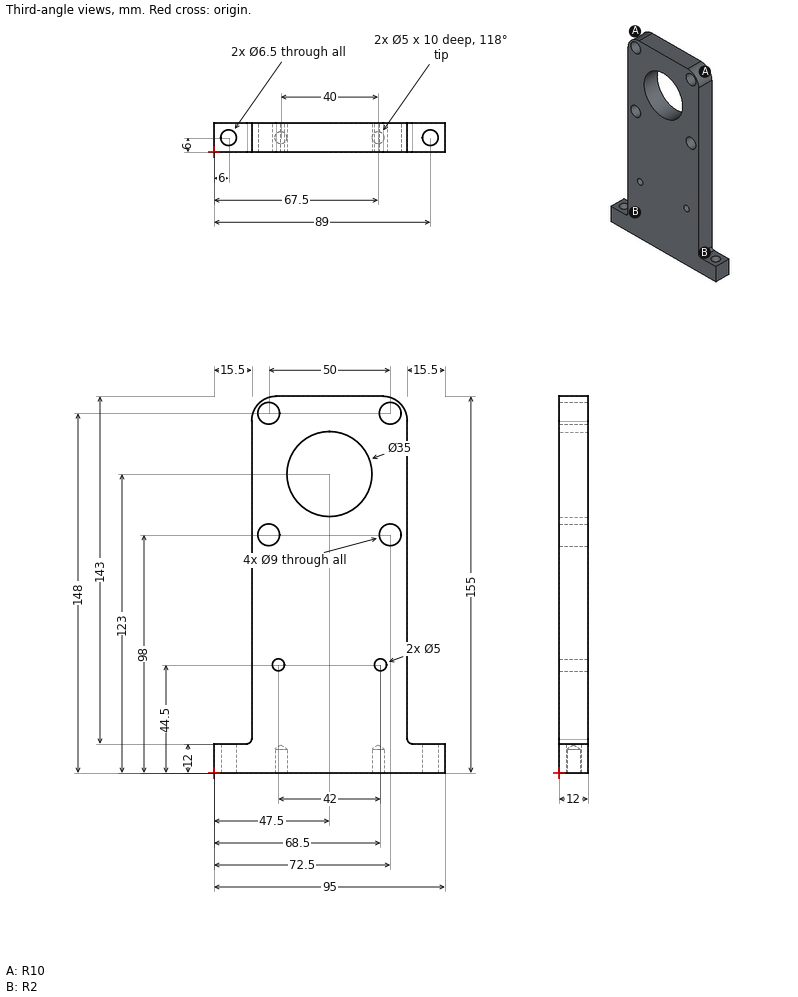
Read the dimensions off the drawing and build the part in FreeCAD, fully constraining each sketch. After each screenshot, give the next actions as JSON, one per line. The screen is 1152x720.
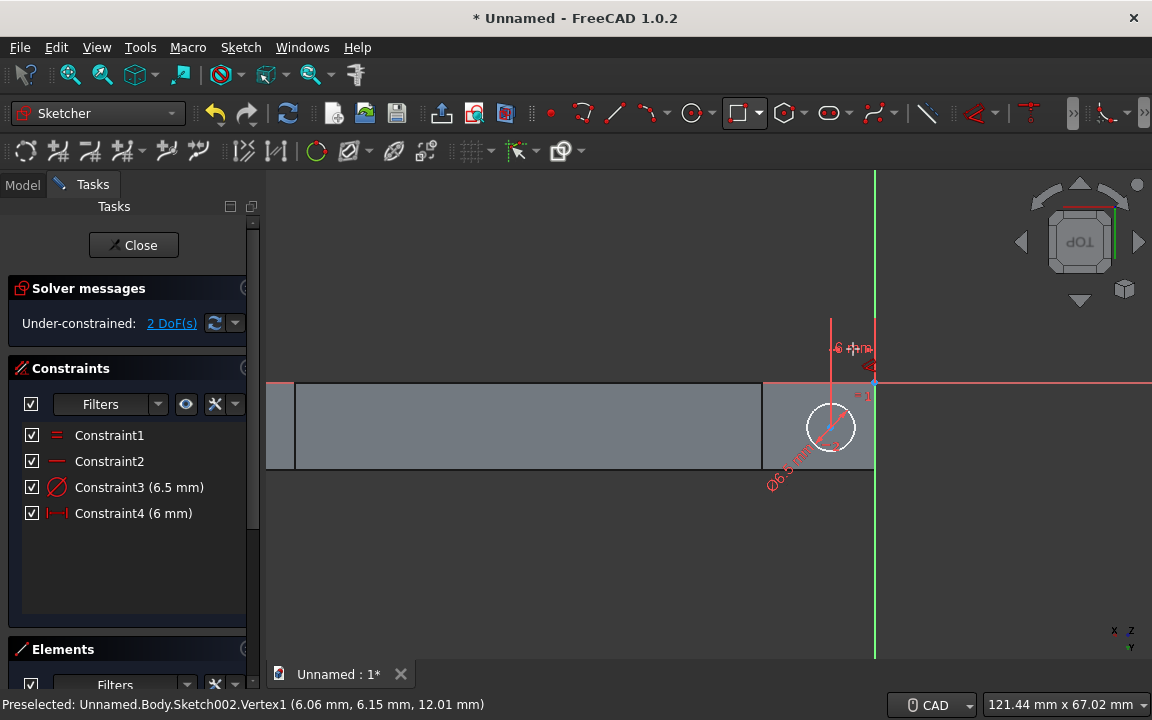
{"action": "left_click", "coordinate": [831, 427]}
{"action": "left_click", "coordinate": [909, 405]}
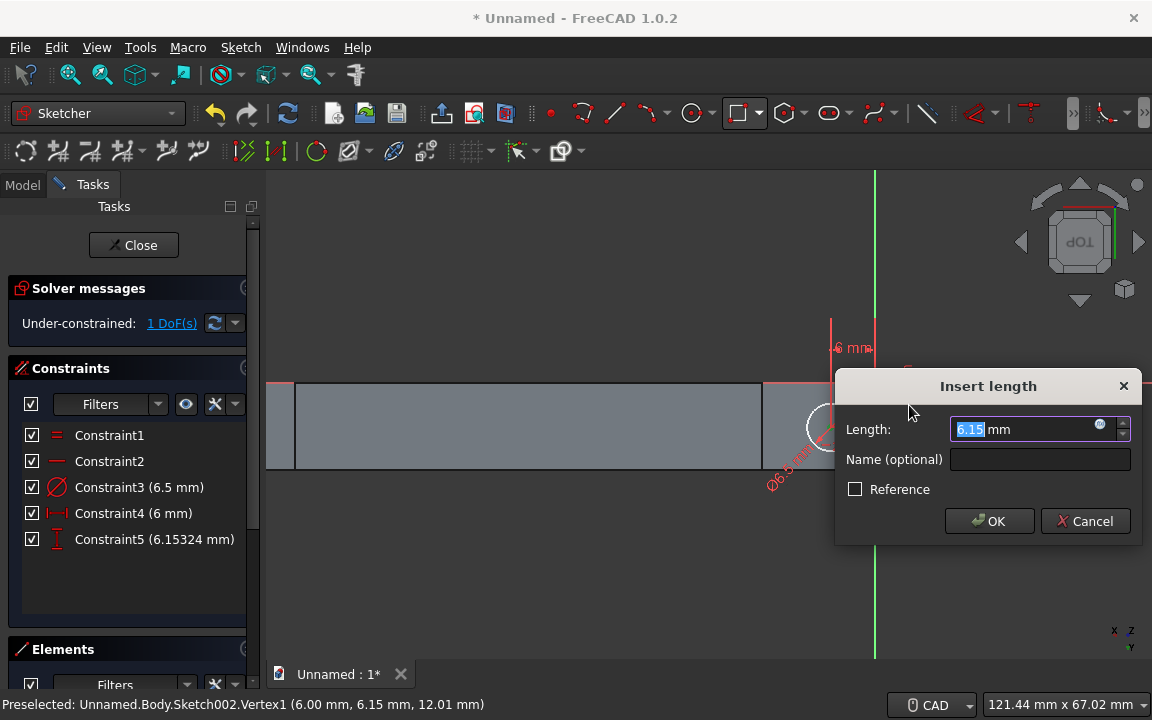
{"action": "type", "text": "6"}
{"action": "key", "text": "Return"}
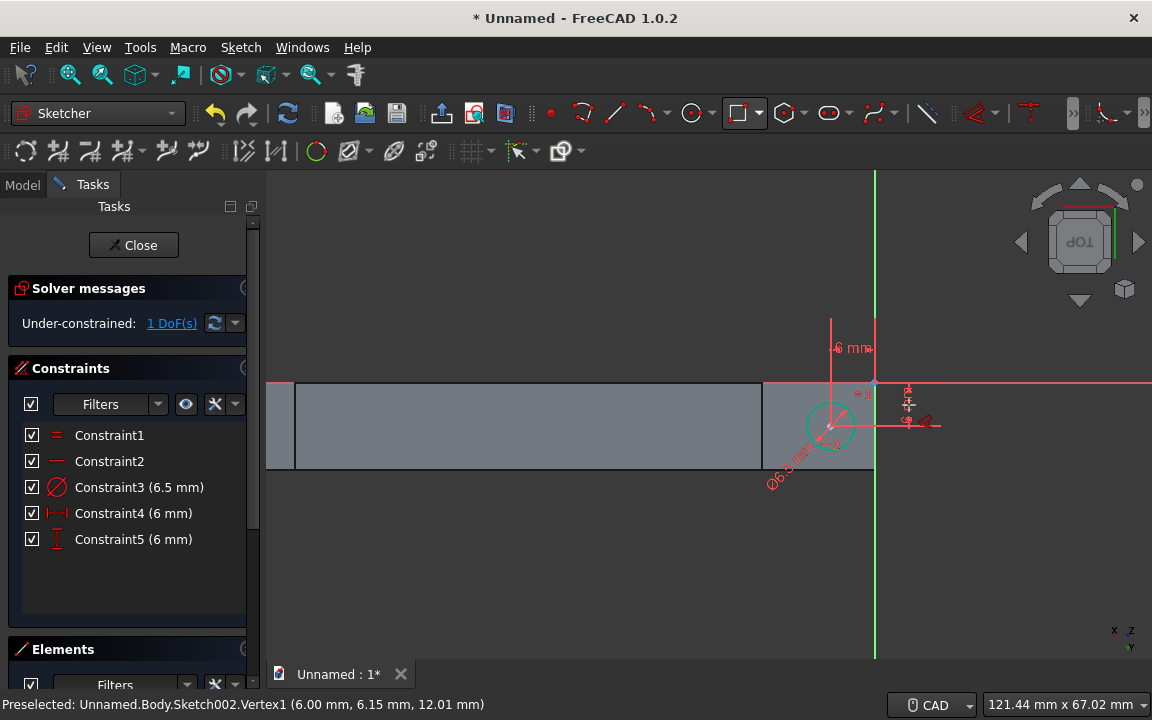
{"action": "scroll", "coordinate": [848, 411], "scroll_direction": "down", "scroll_amount": 2}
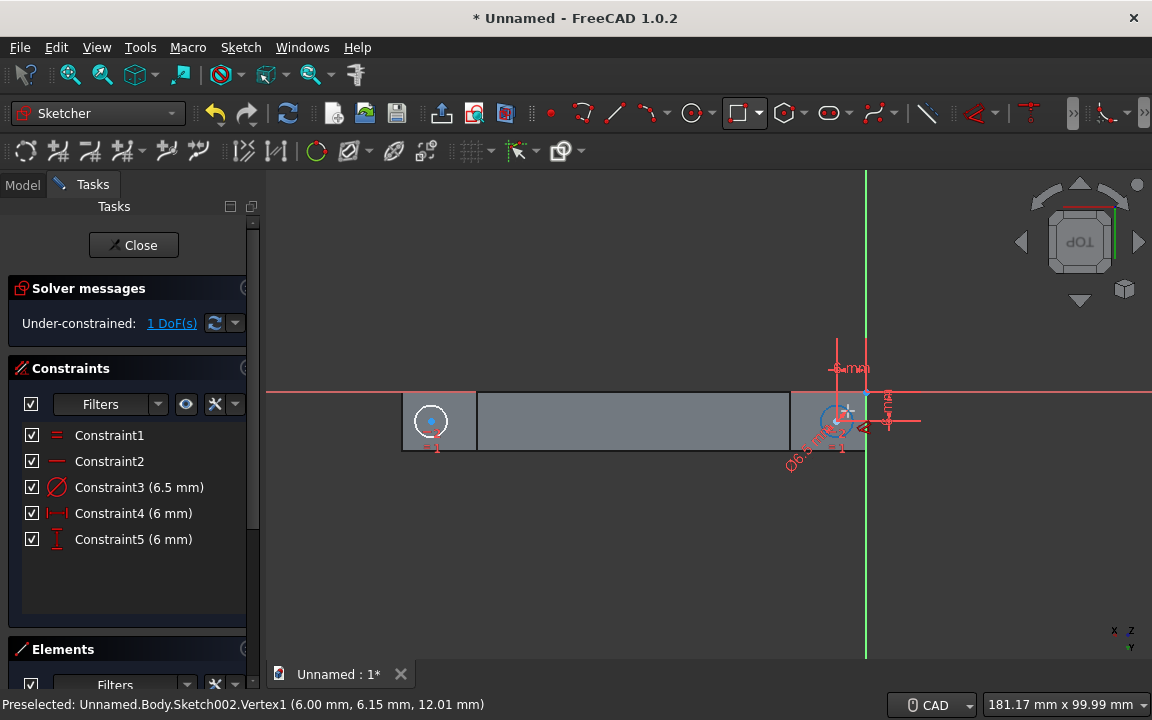
{"action": "left_click", "coordinate": [431, 421]}
{"action": "left_click", "coordinate": [649, 358]}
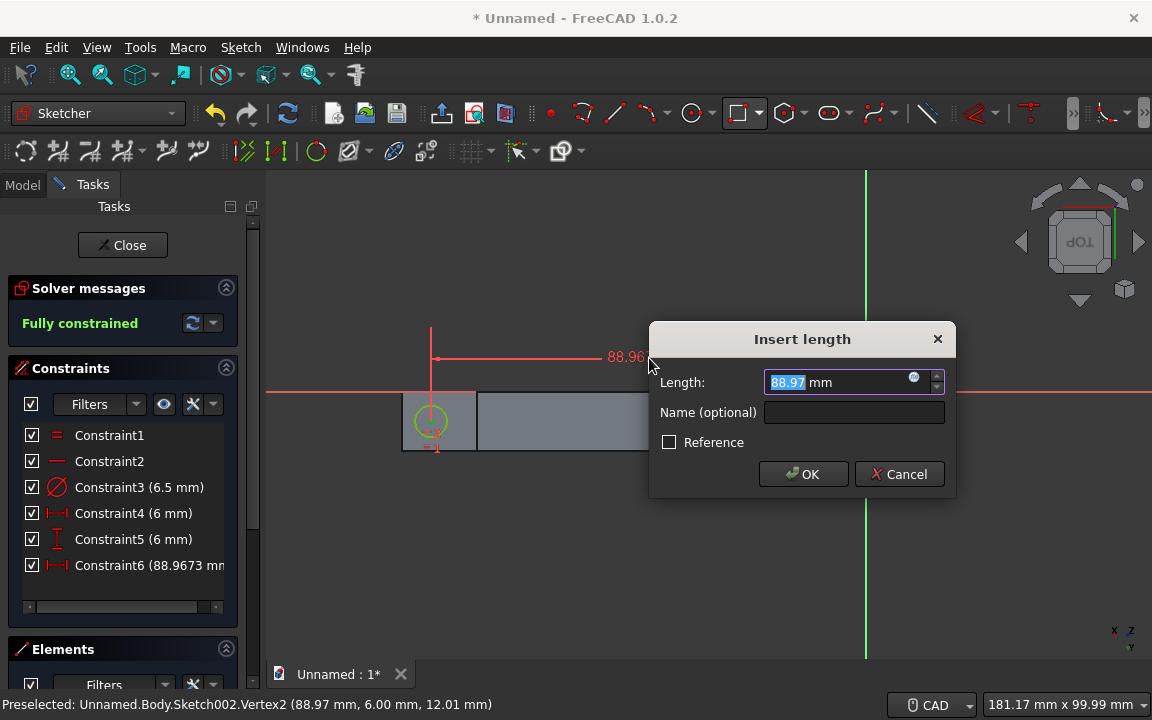
{"action": "type", "text": "89"}
{"action": "key", "text": "Return"}
{"action": "key", "text": "Escape"}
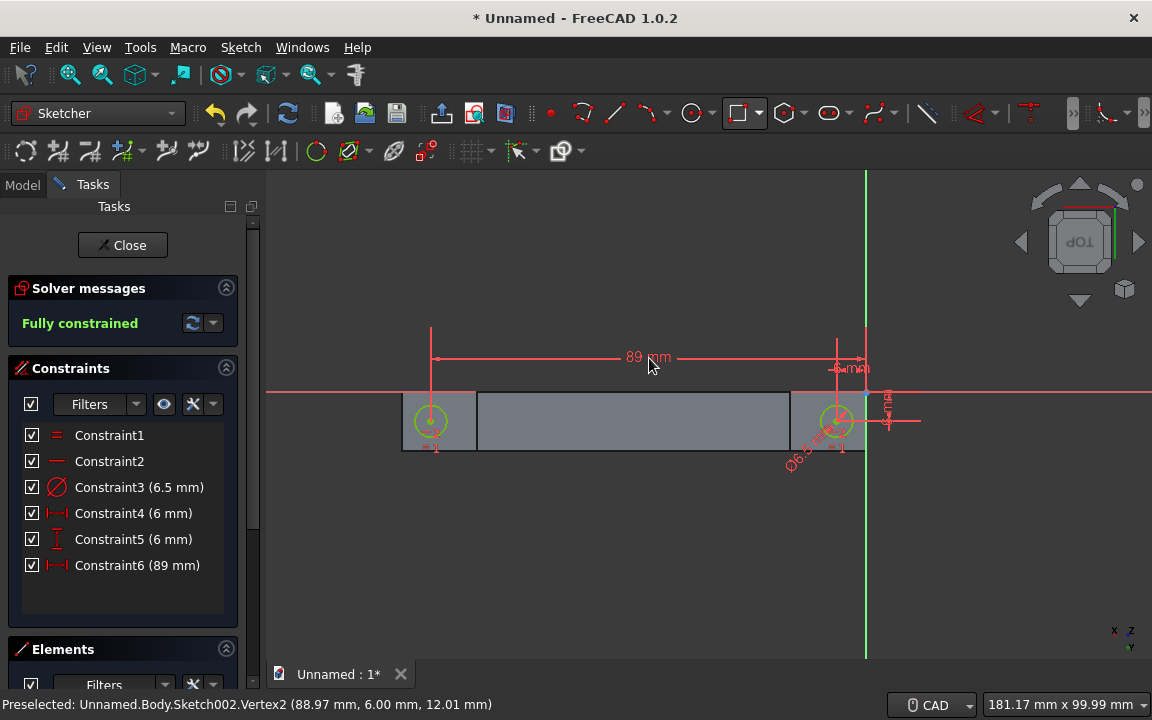
{"action": "left_click", "coordinate": [123, 245]}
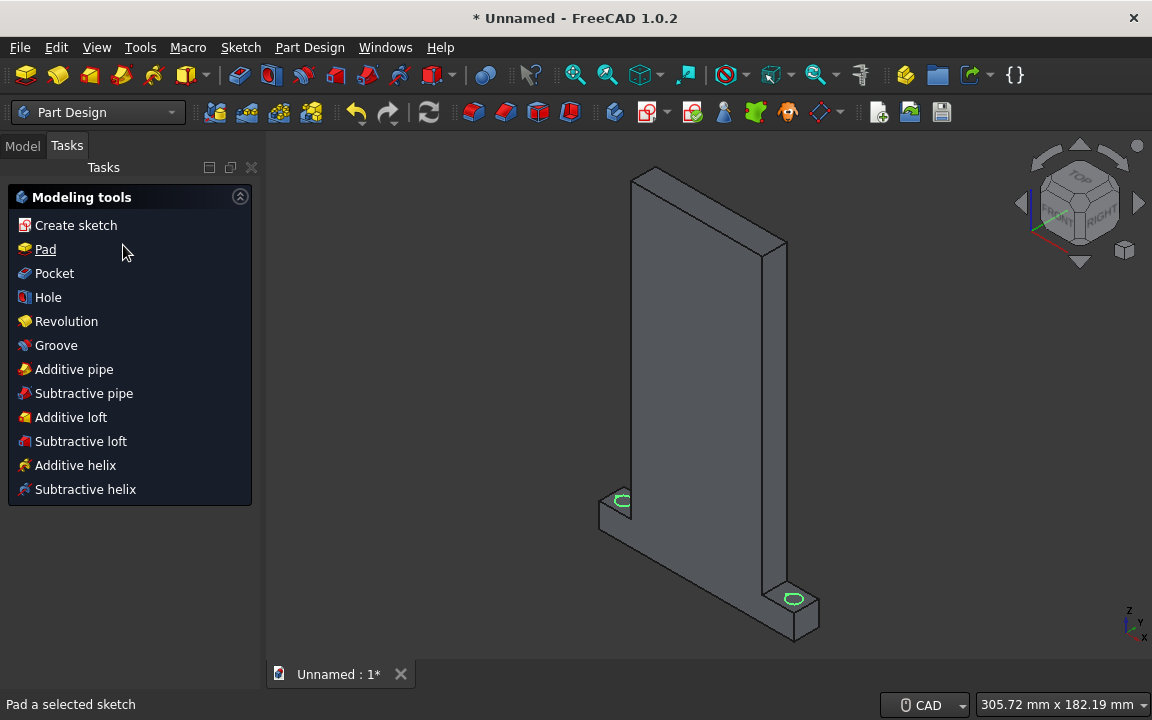
{"action": "left_click", "coordinate": [272, 76]}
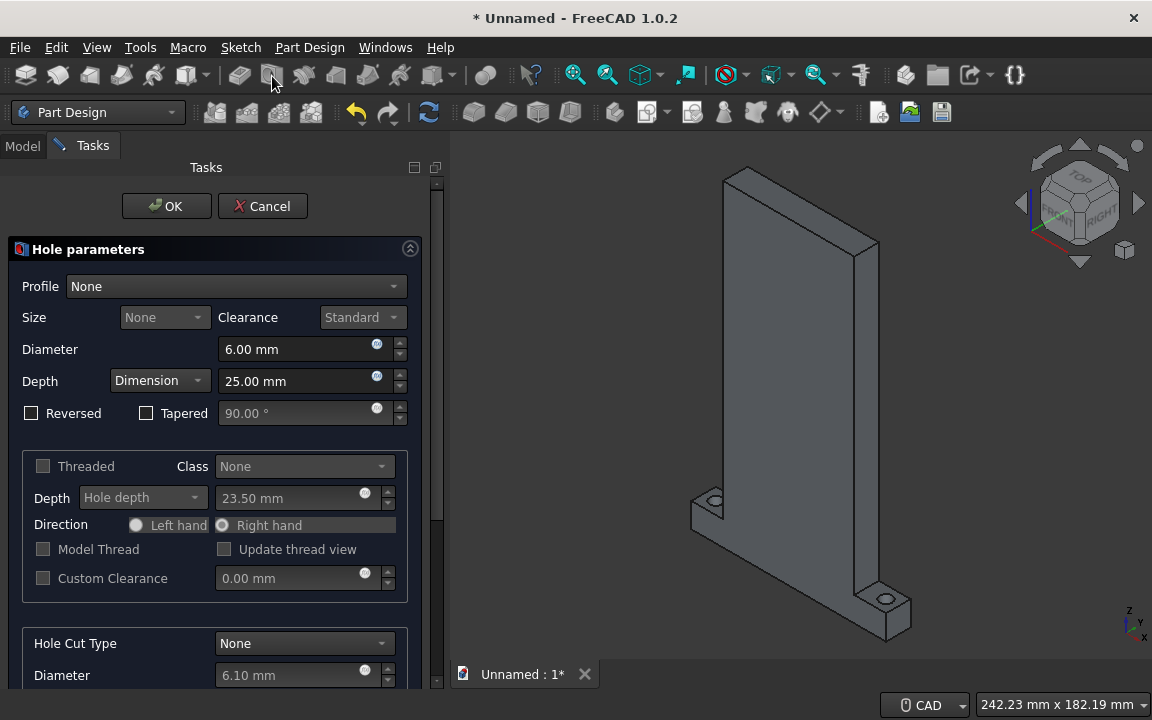
{"action": "triple_click", "coordinate": [305, 349]}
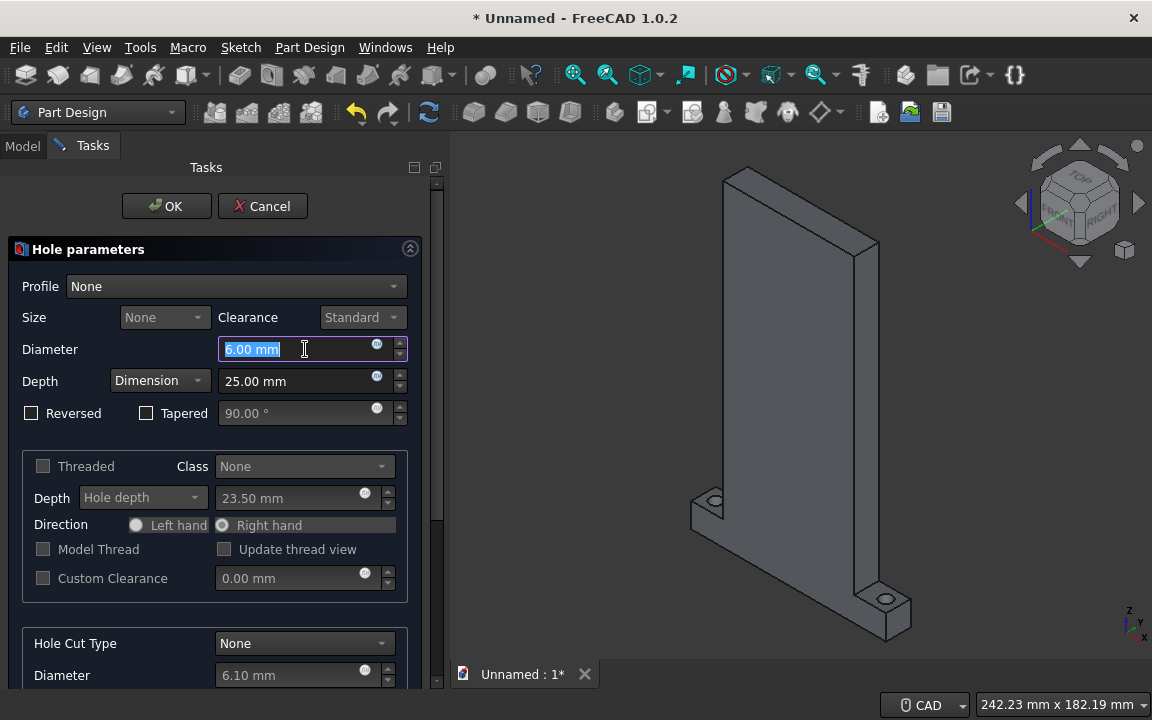
{"action": "type", "text": "6.5"}
{"action": "key", "text": "Tab"}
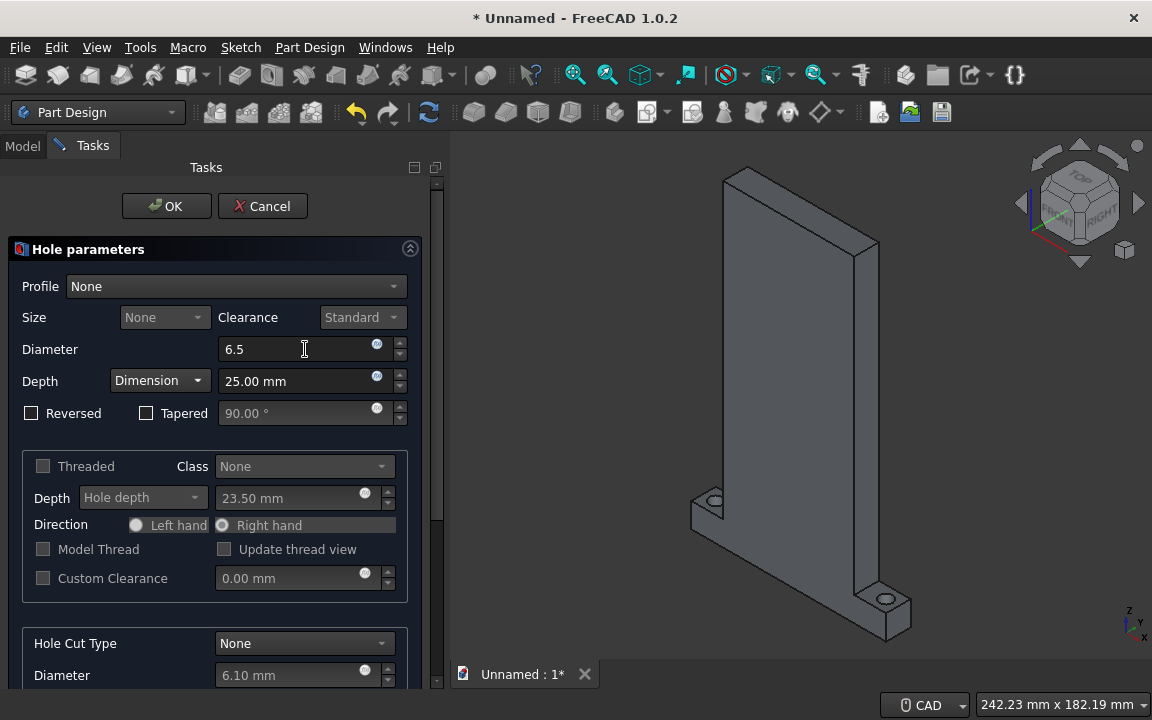
{"action": "left_click", "coordinate": [161, 380]}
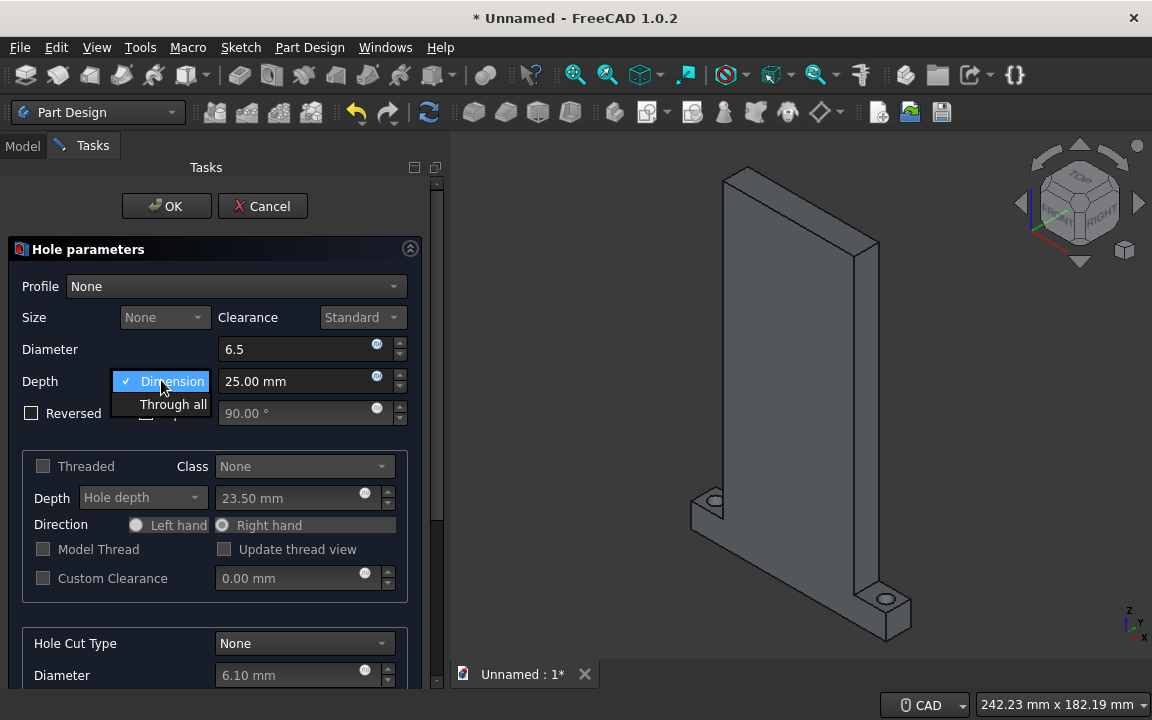
{"action": "left_click", "coordinate": [160, 404]}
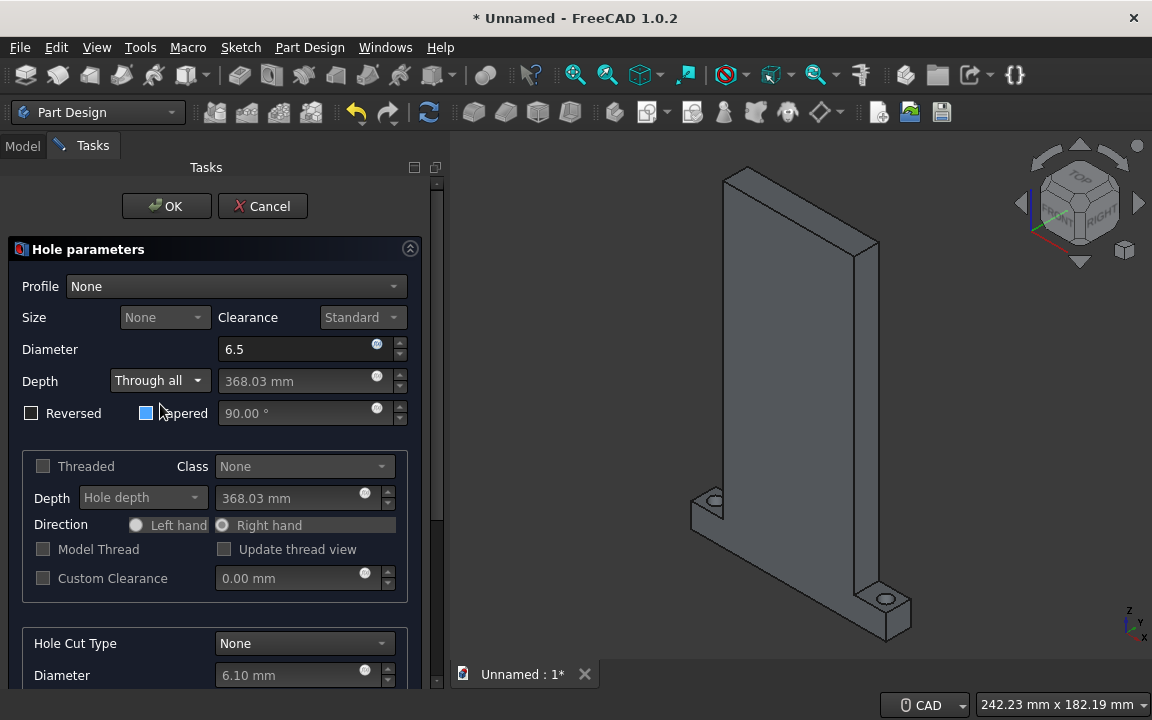
{"action": "left_click", "coordinate": [167, 206]}